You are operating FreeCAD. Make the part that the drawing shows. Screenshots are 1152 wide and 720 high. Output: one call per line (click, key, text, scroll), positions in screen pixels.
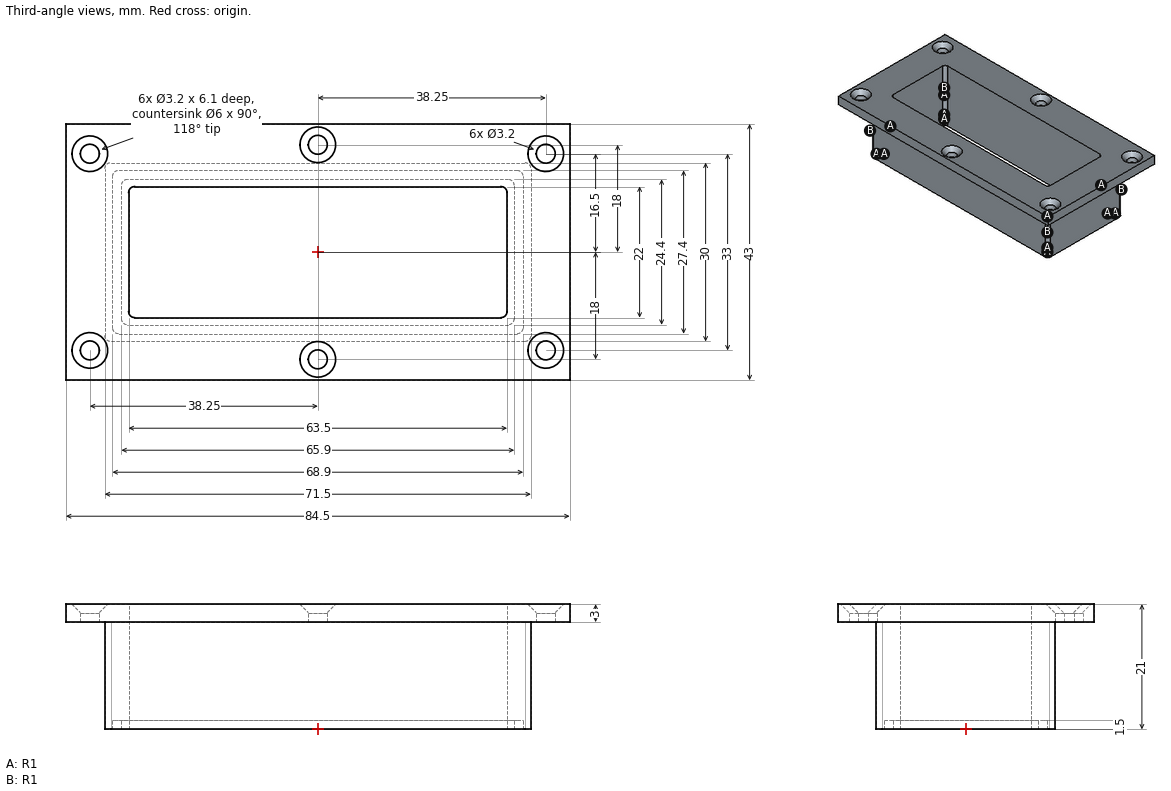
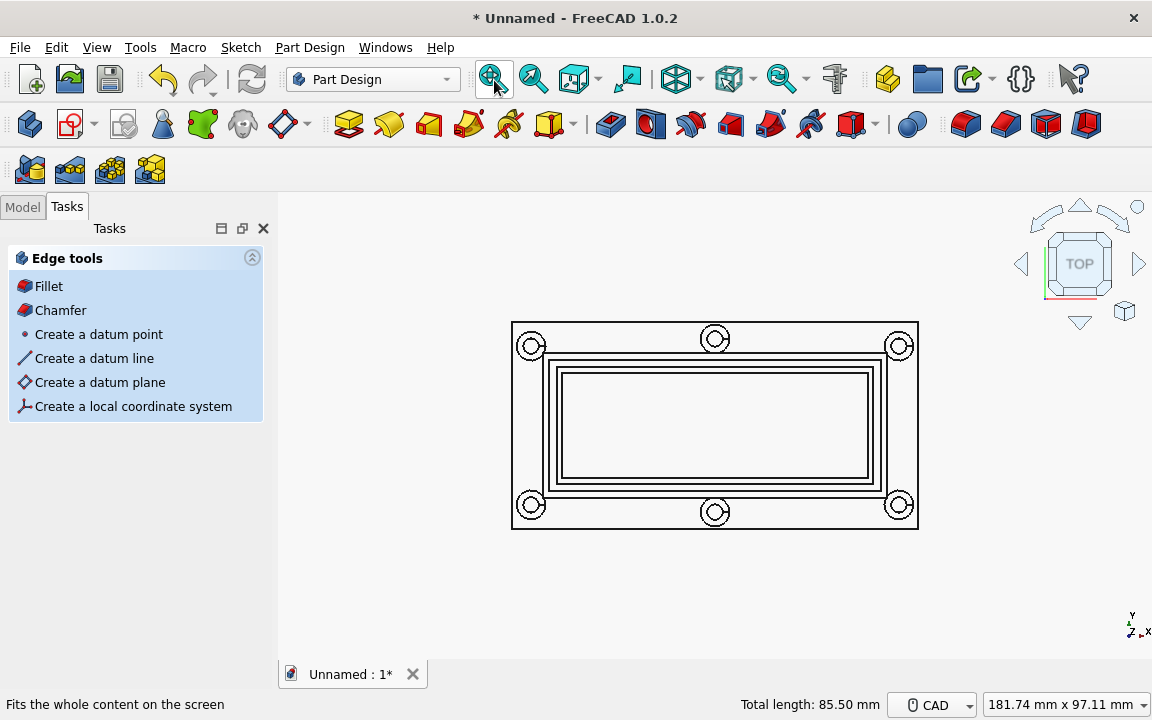
scroll(881, 359, up, 9)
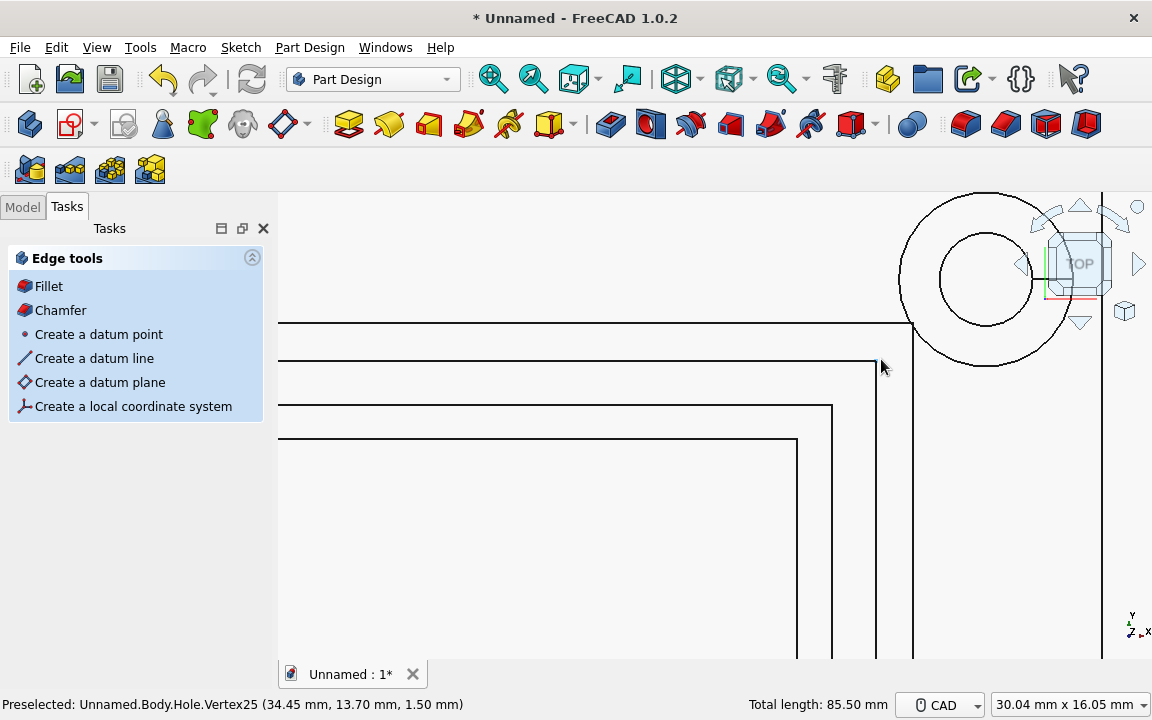
click(494, 80)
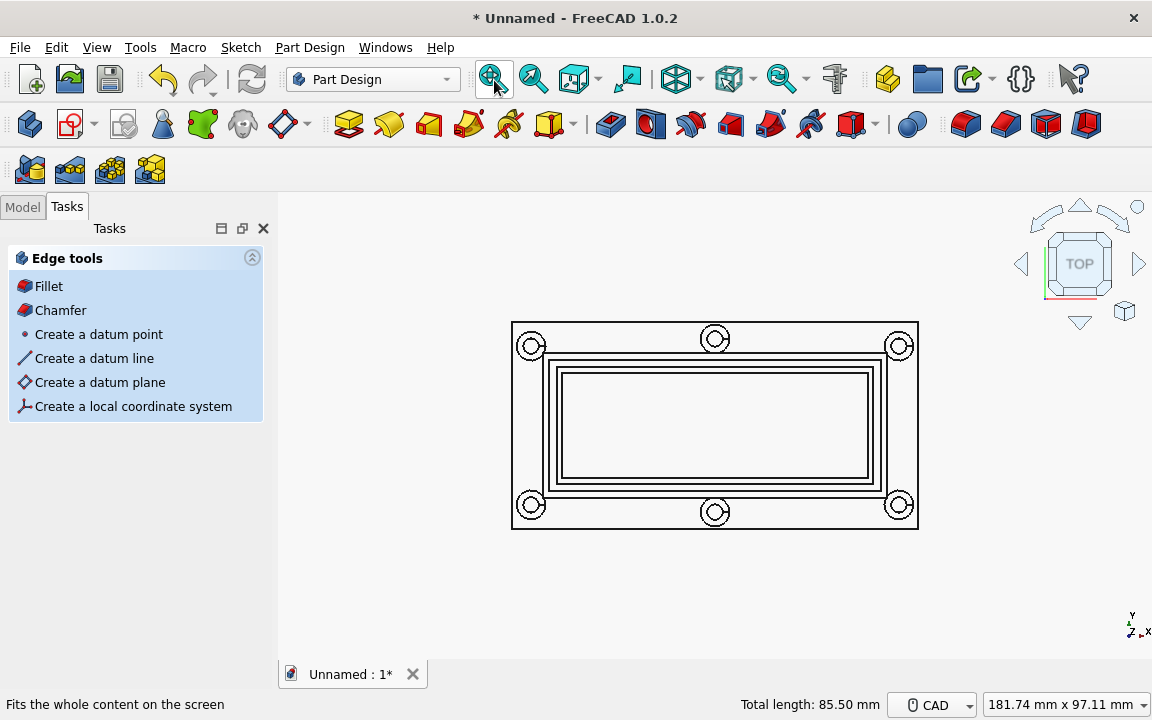
key(1)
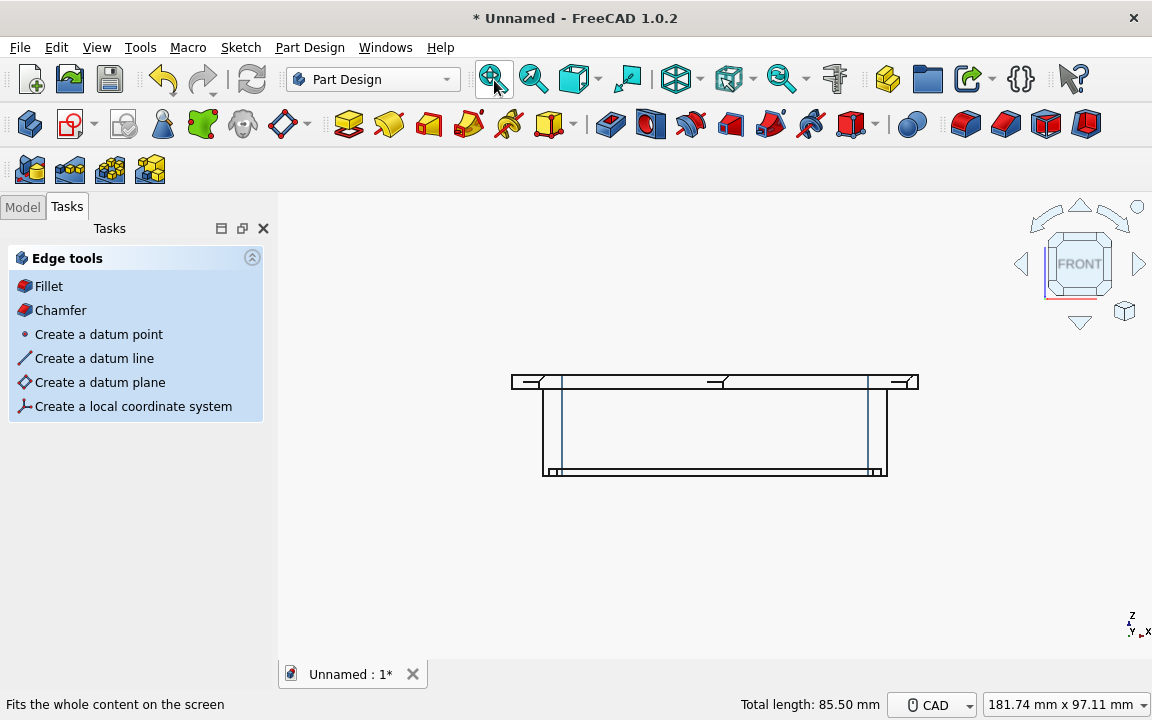
scroll(881, 471, up, 9)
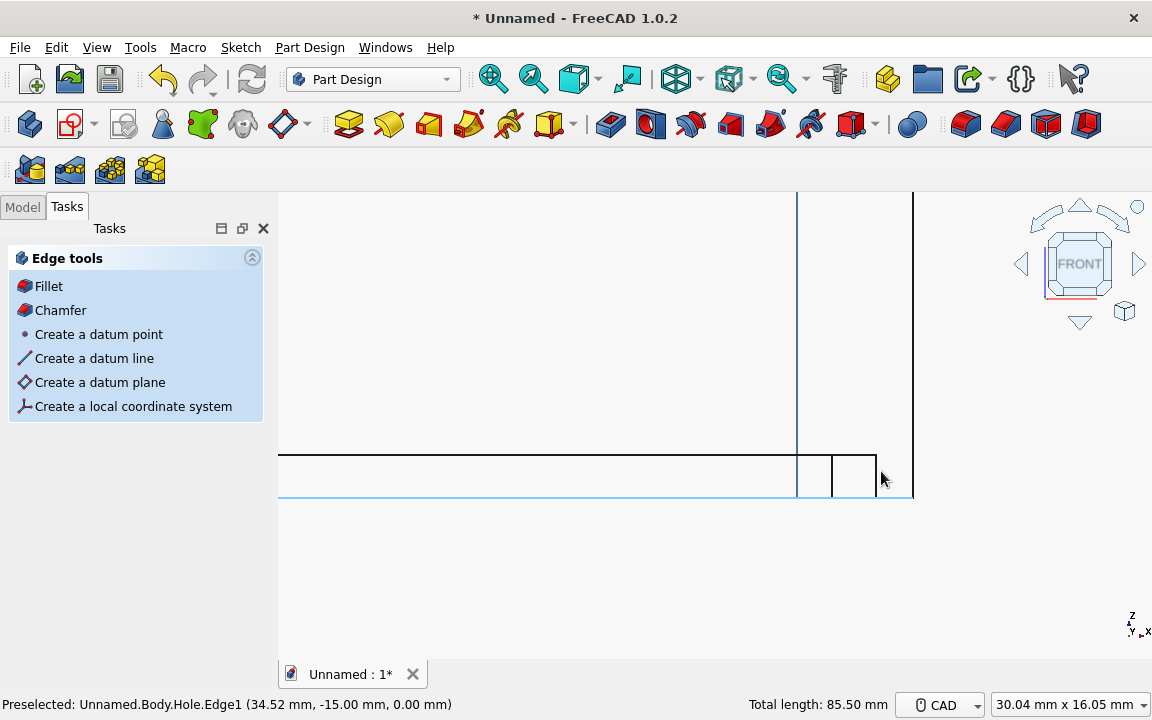
click(876, 475, ctrl)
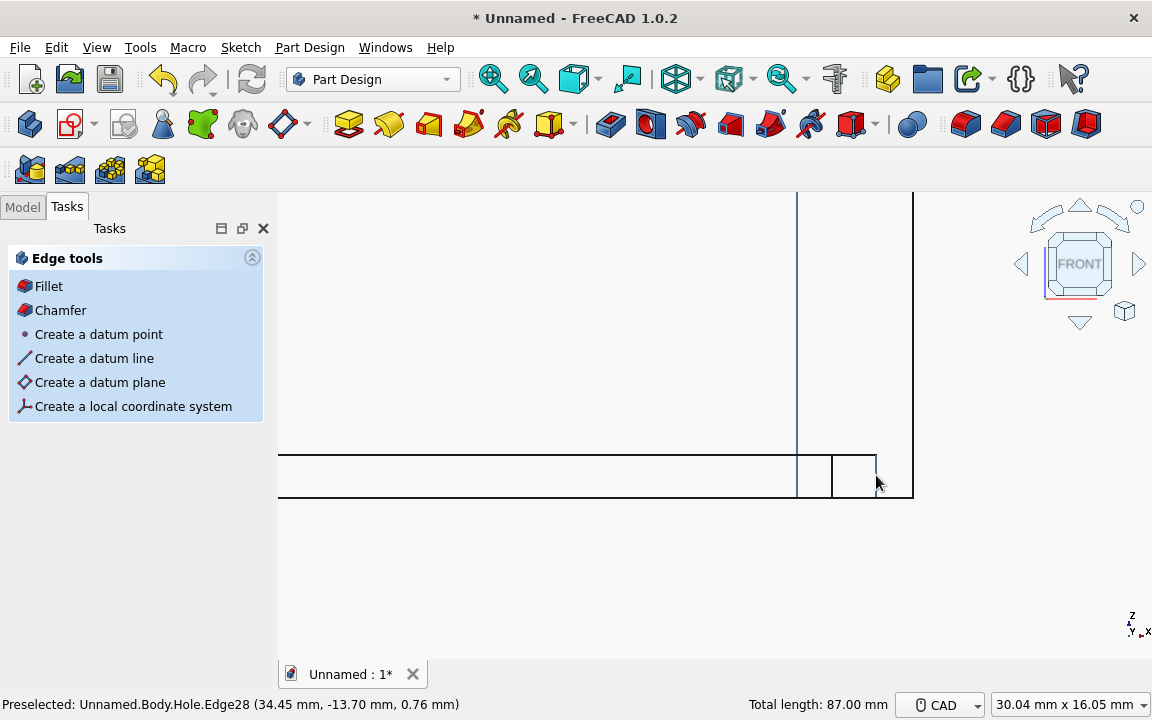
click(832, 475, ctrl)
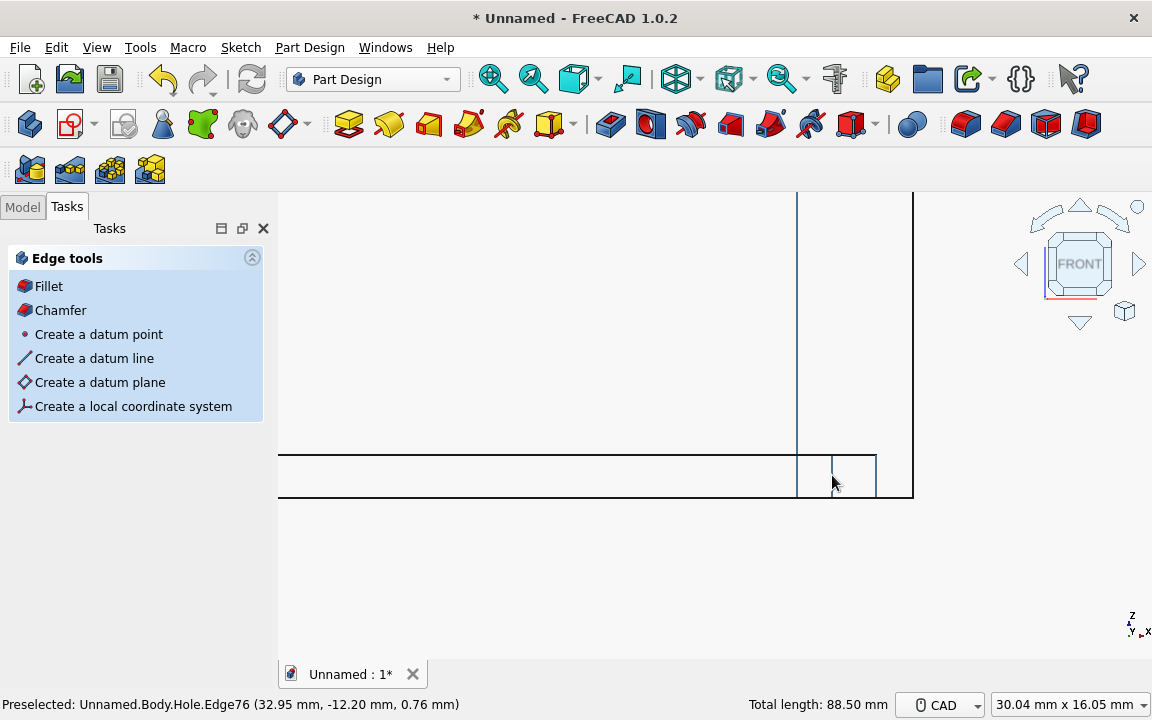
click(494, 80)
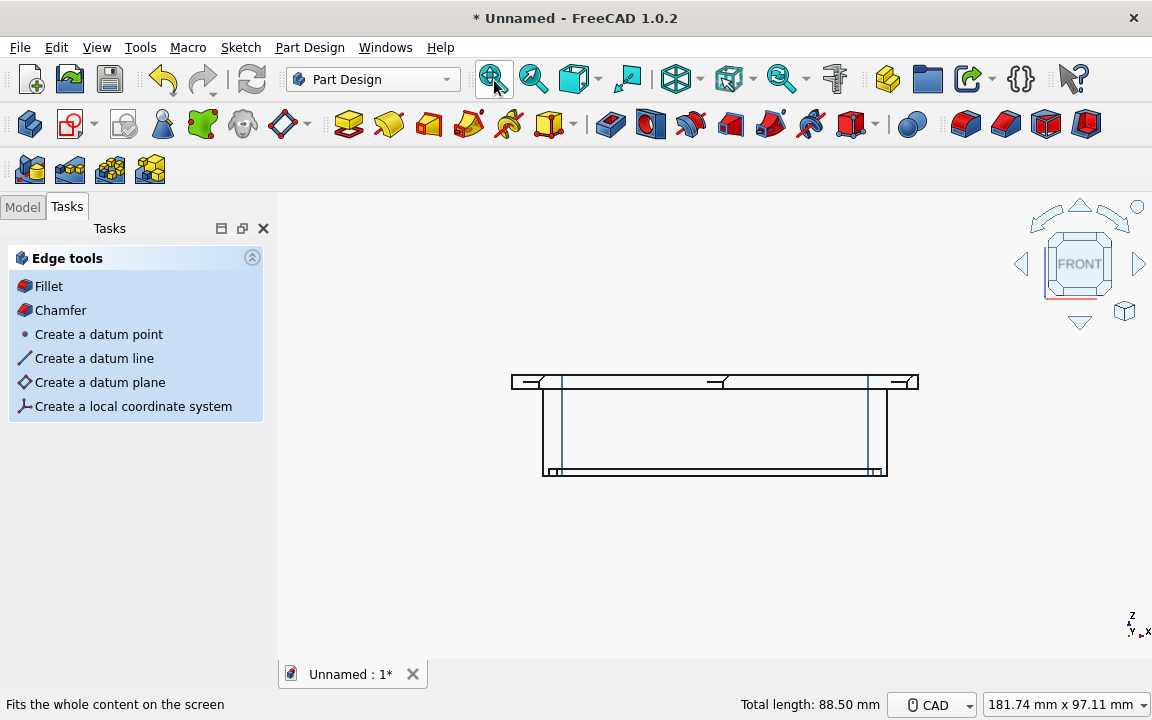
key(3)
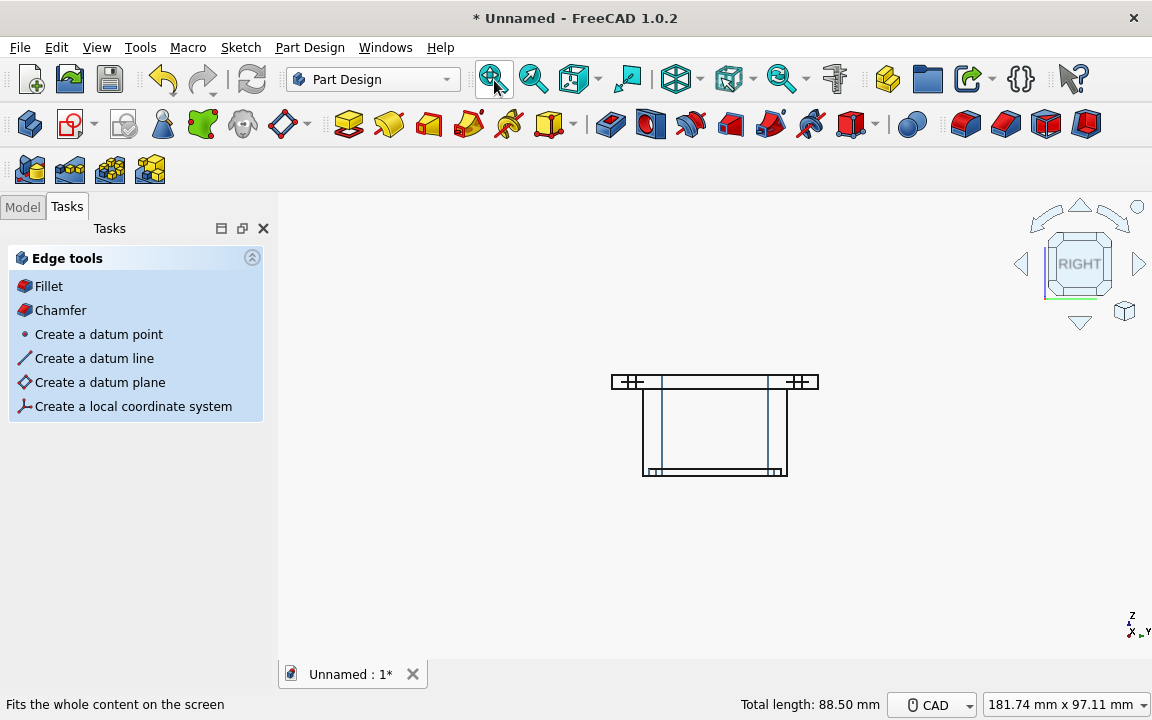
click(494, 80)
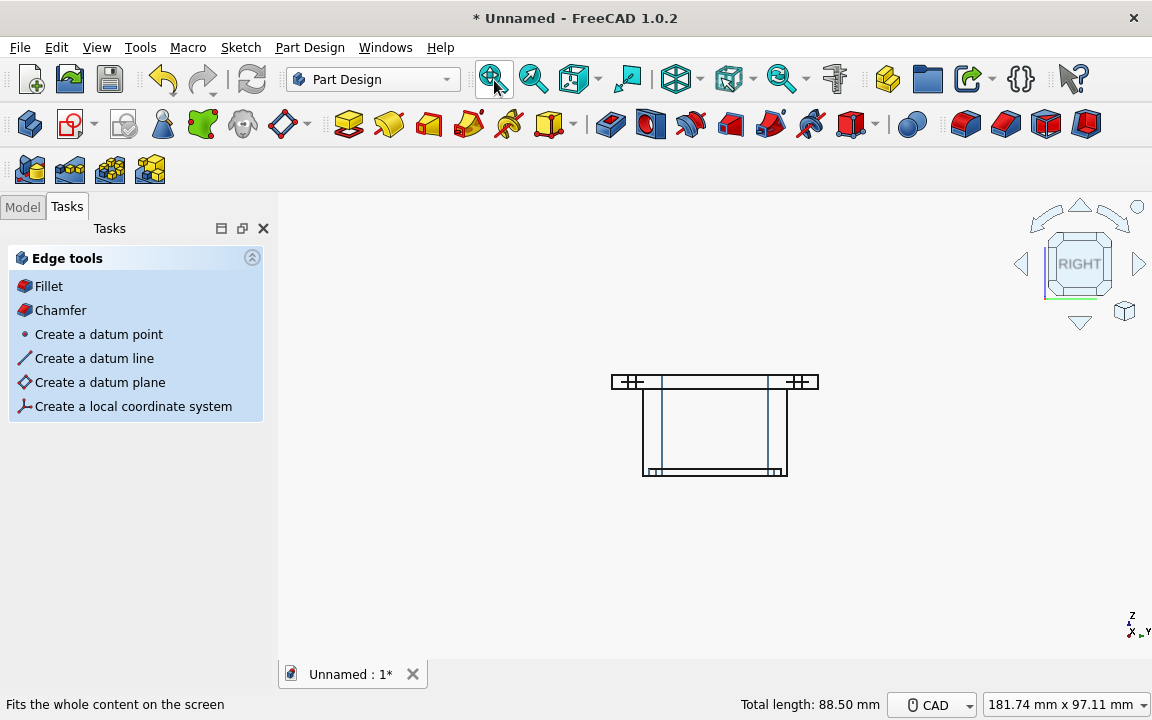
scroll(781, 471, up, 9)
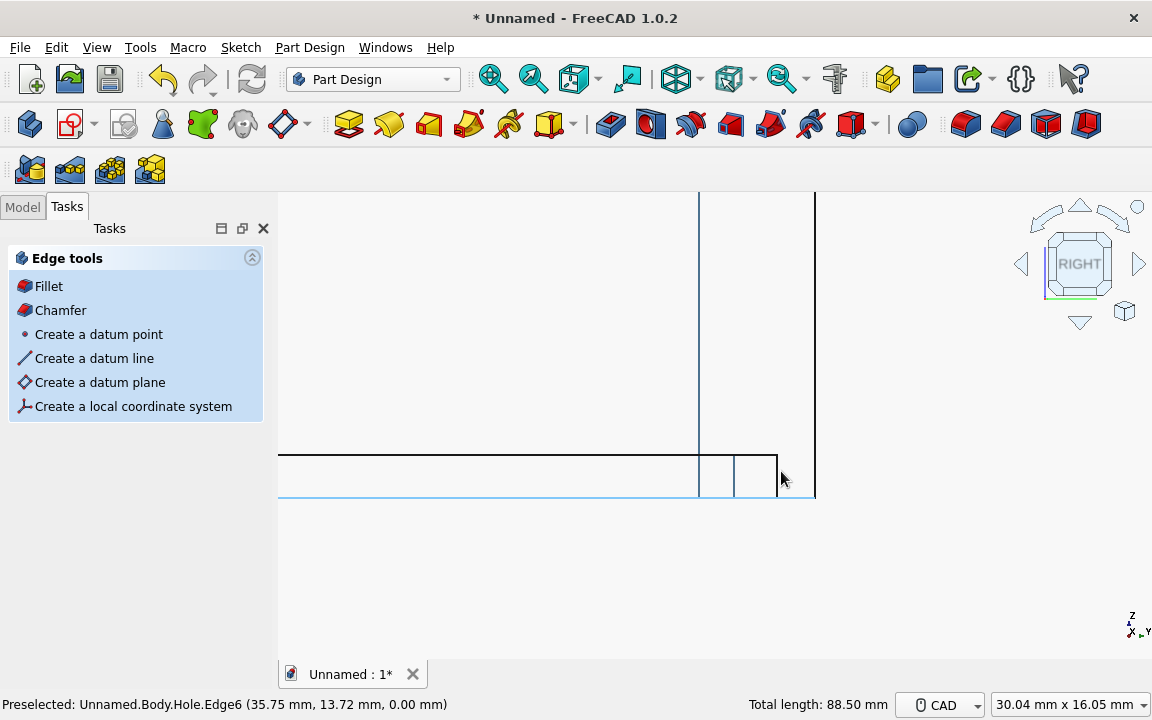
click(777, 475, ctrl)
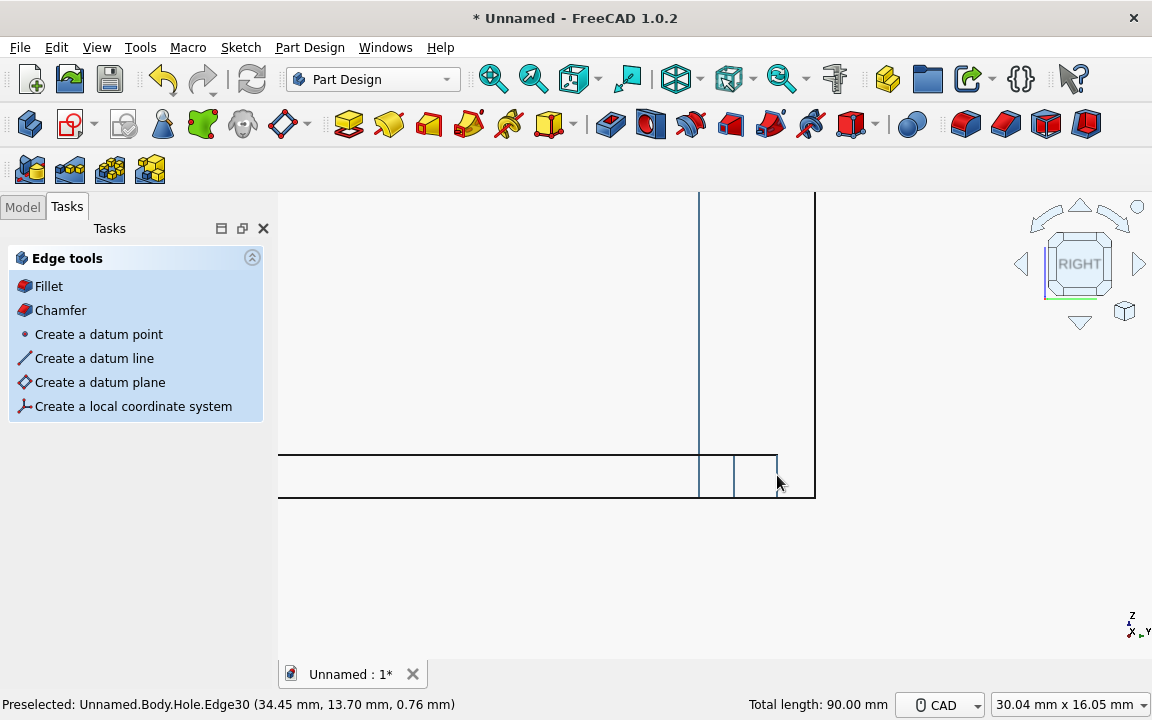
click(494, 80)